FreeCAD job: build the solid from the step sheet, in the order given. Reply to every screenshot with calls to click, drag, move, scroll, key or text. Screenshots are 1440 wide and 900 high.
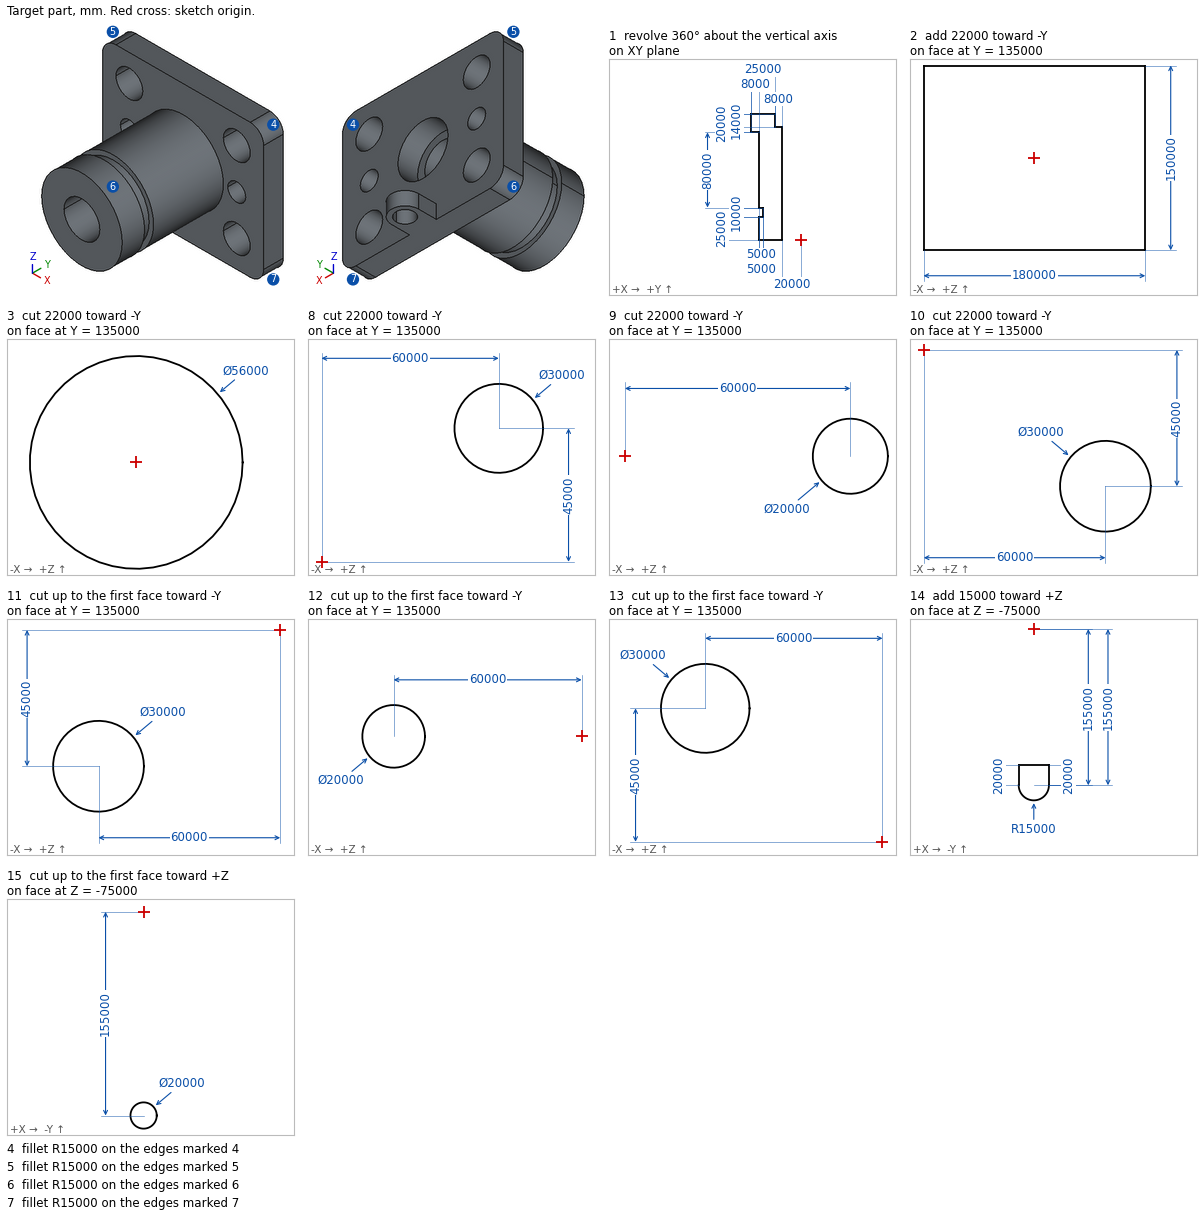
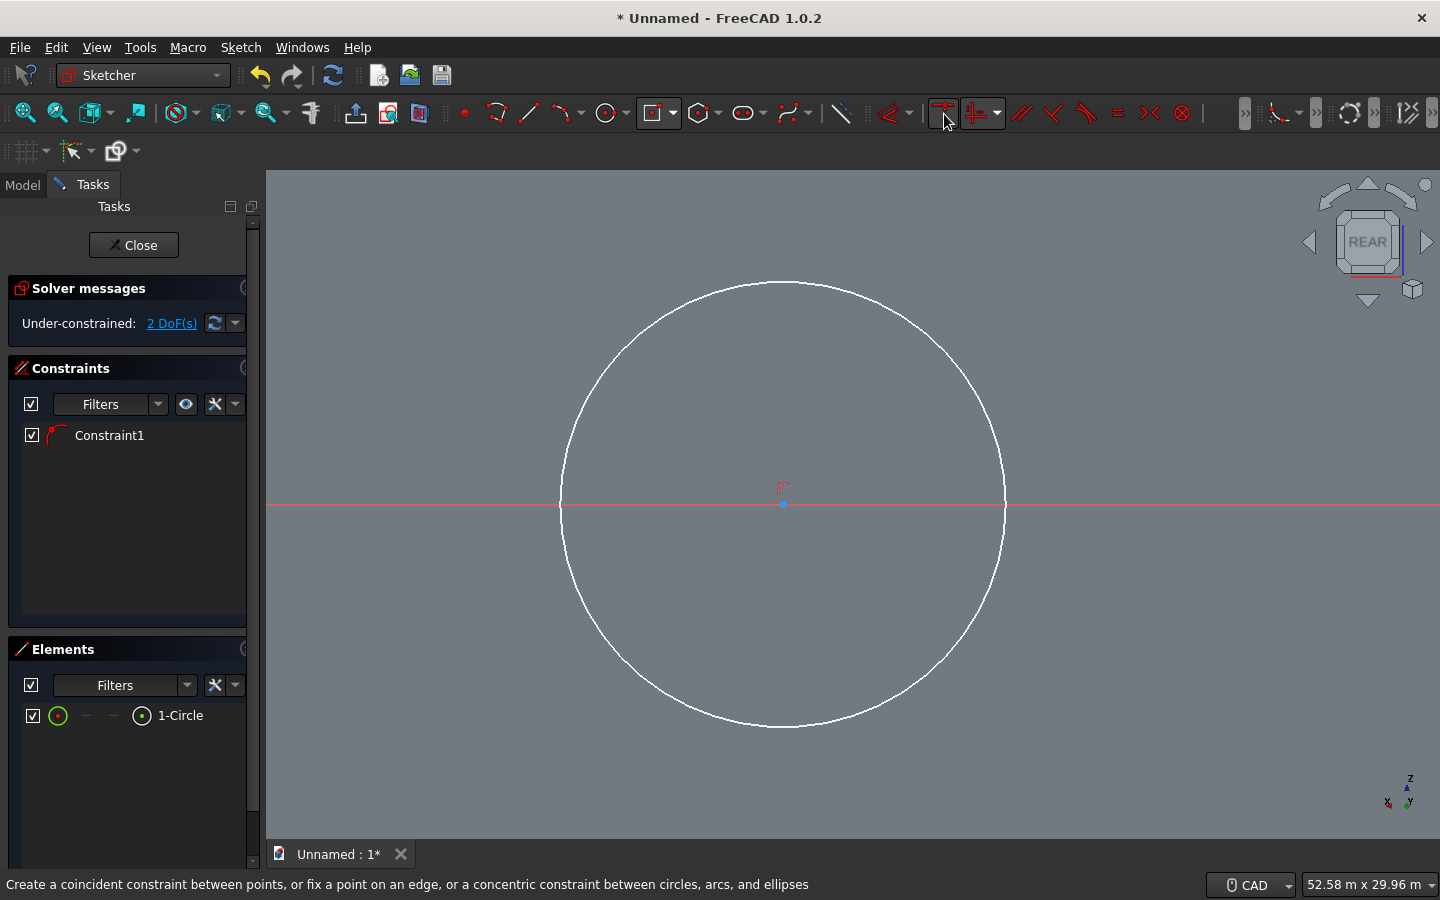
click(940, 347)
click(963, 324)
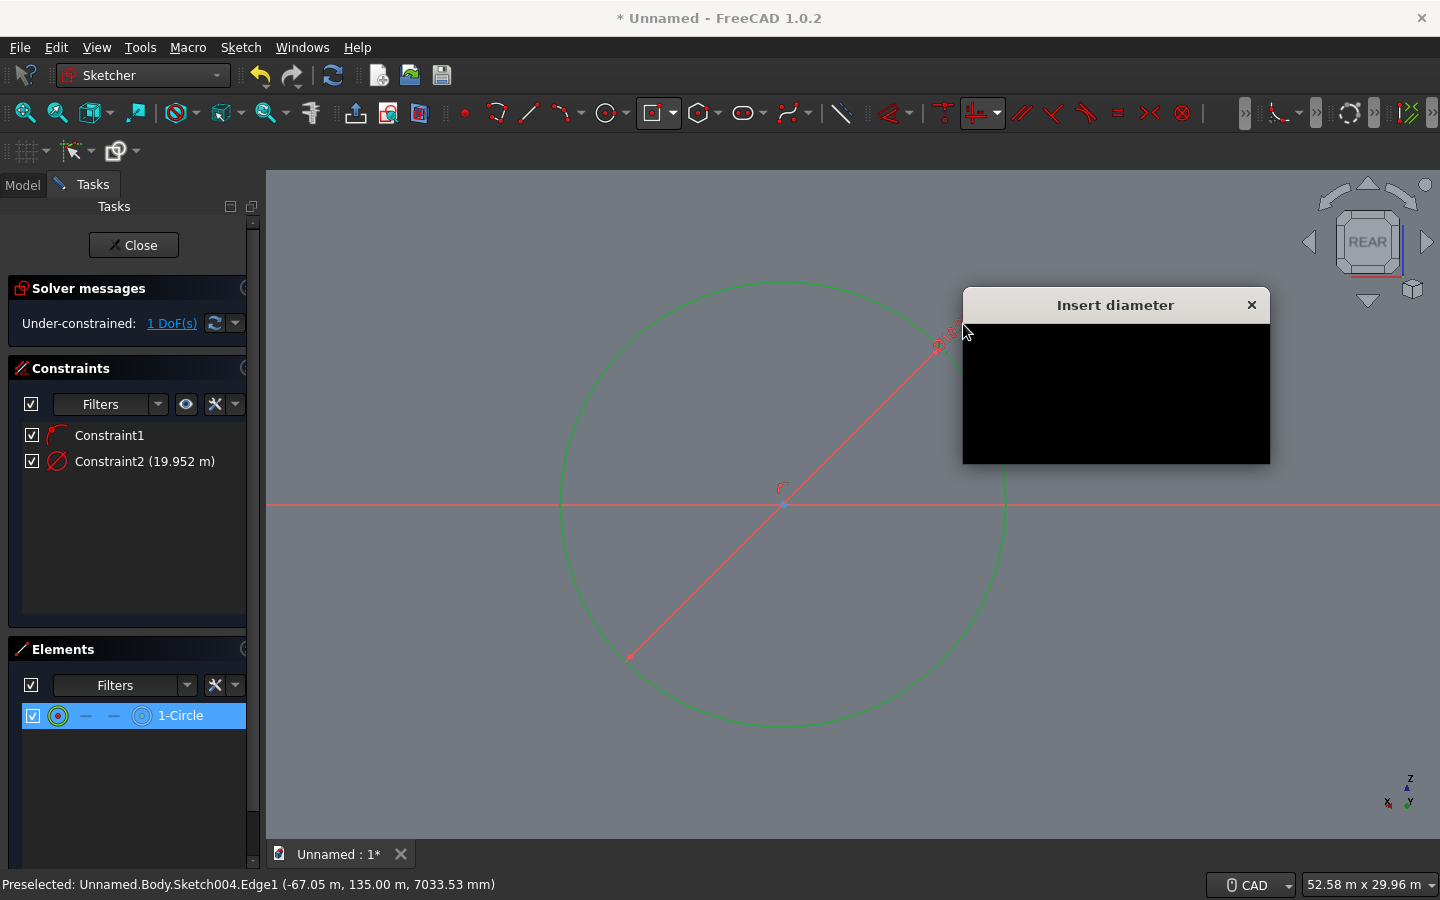
key(ctrl+a)
text(20000 mm)
key(Return)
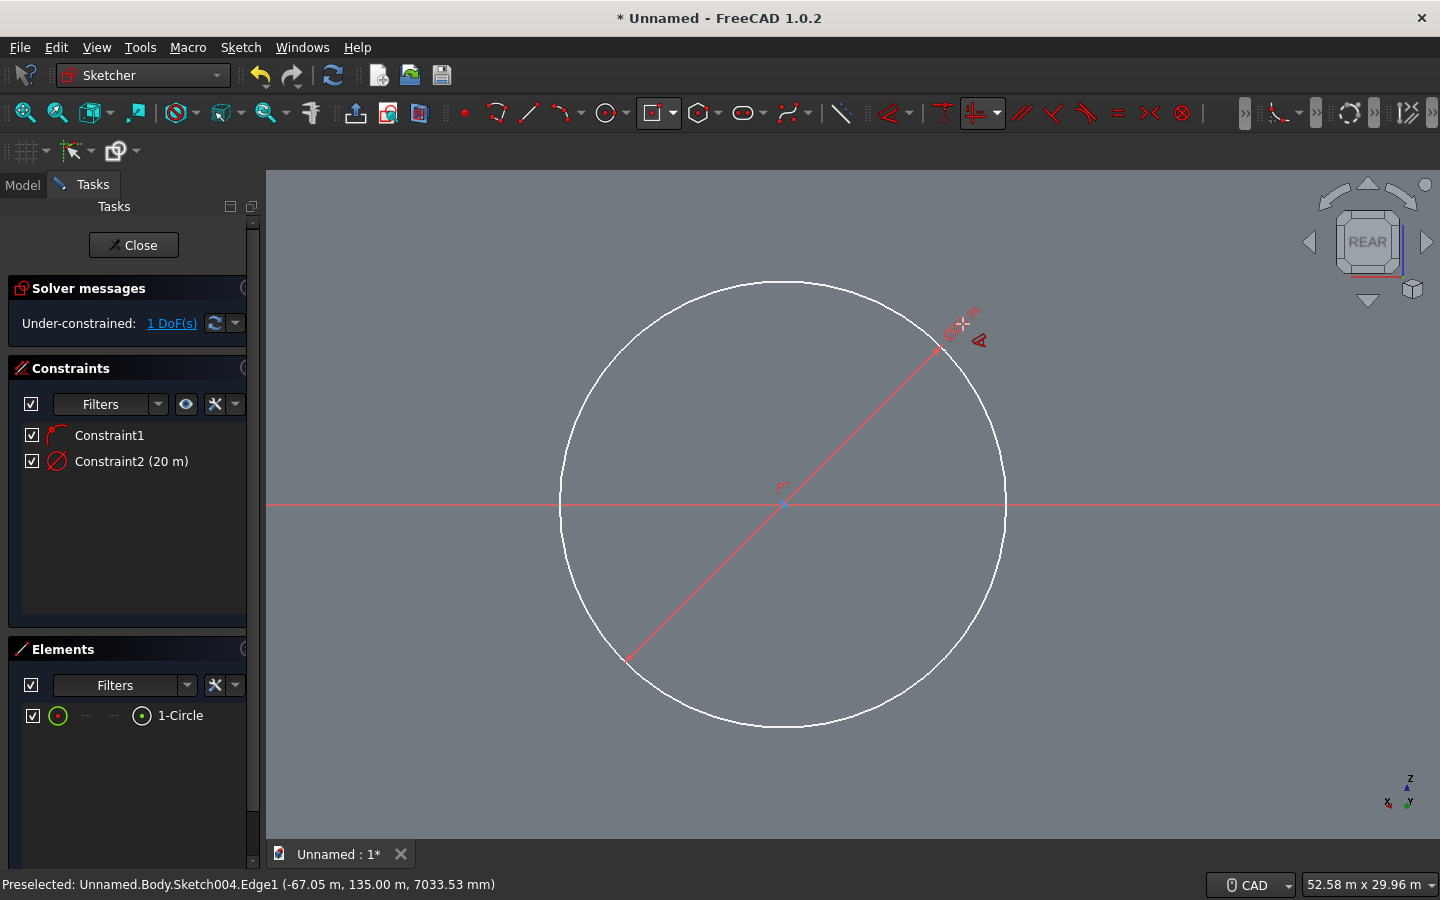
click(783, 504)
click(539, 538)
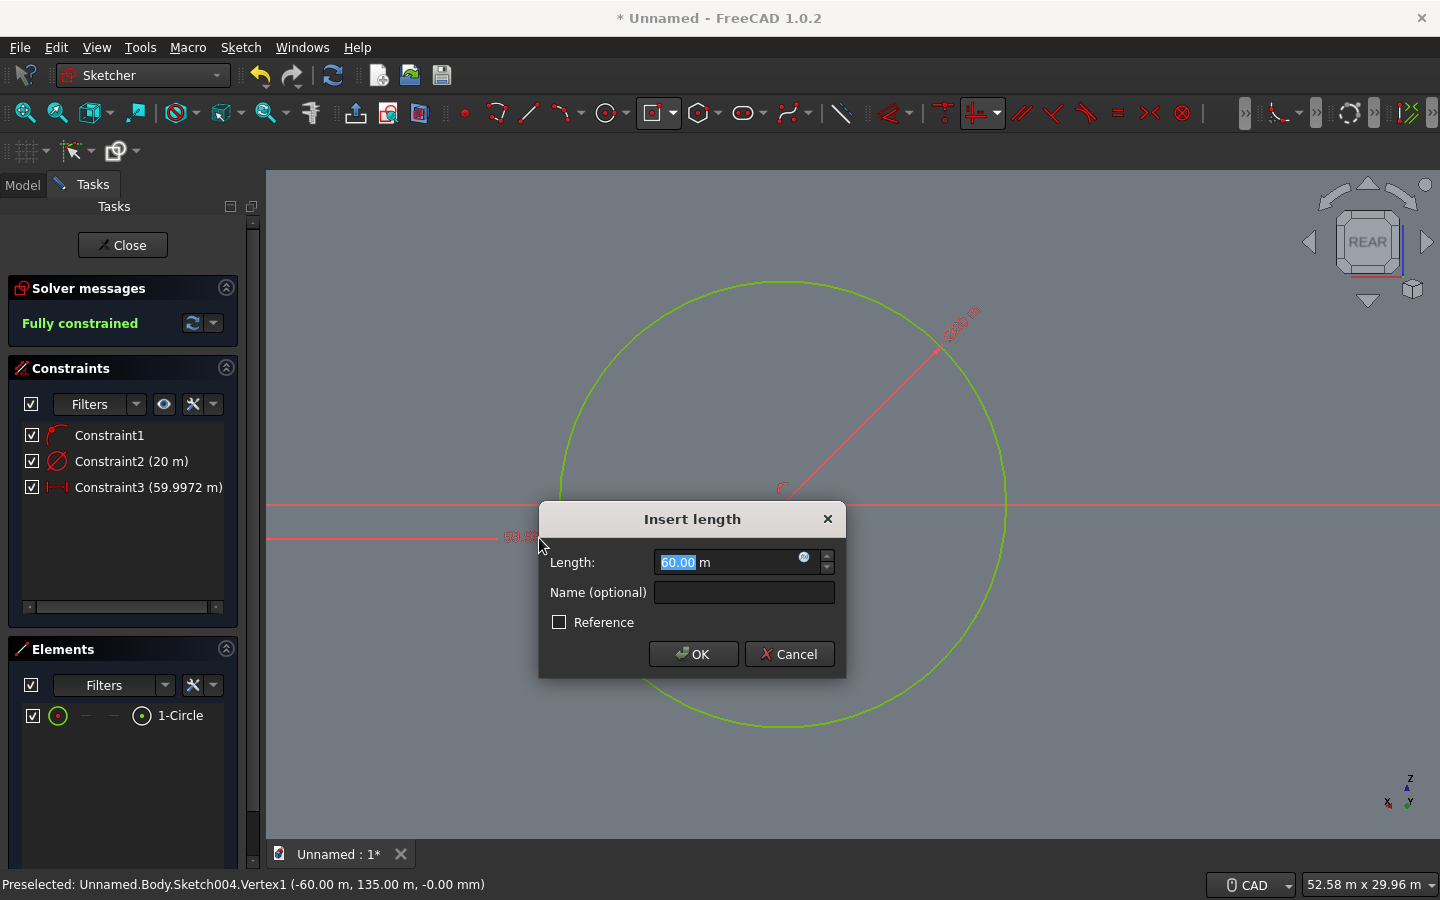
key(ctrl+a)
text(60000 mm)
key(Return)
key(Escape)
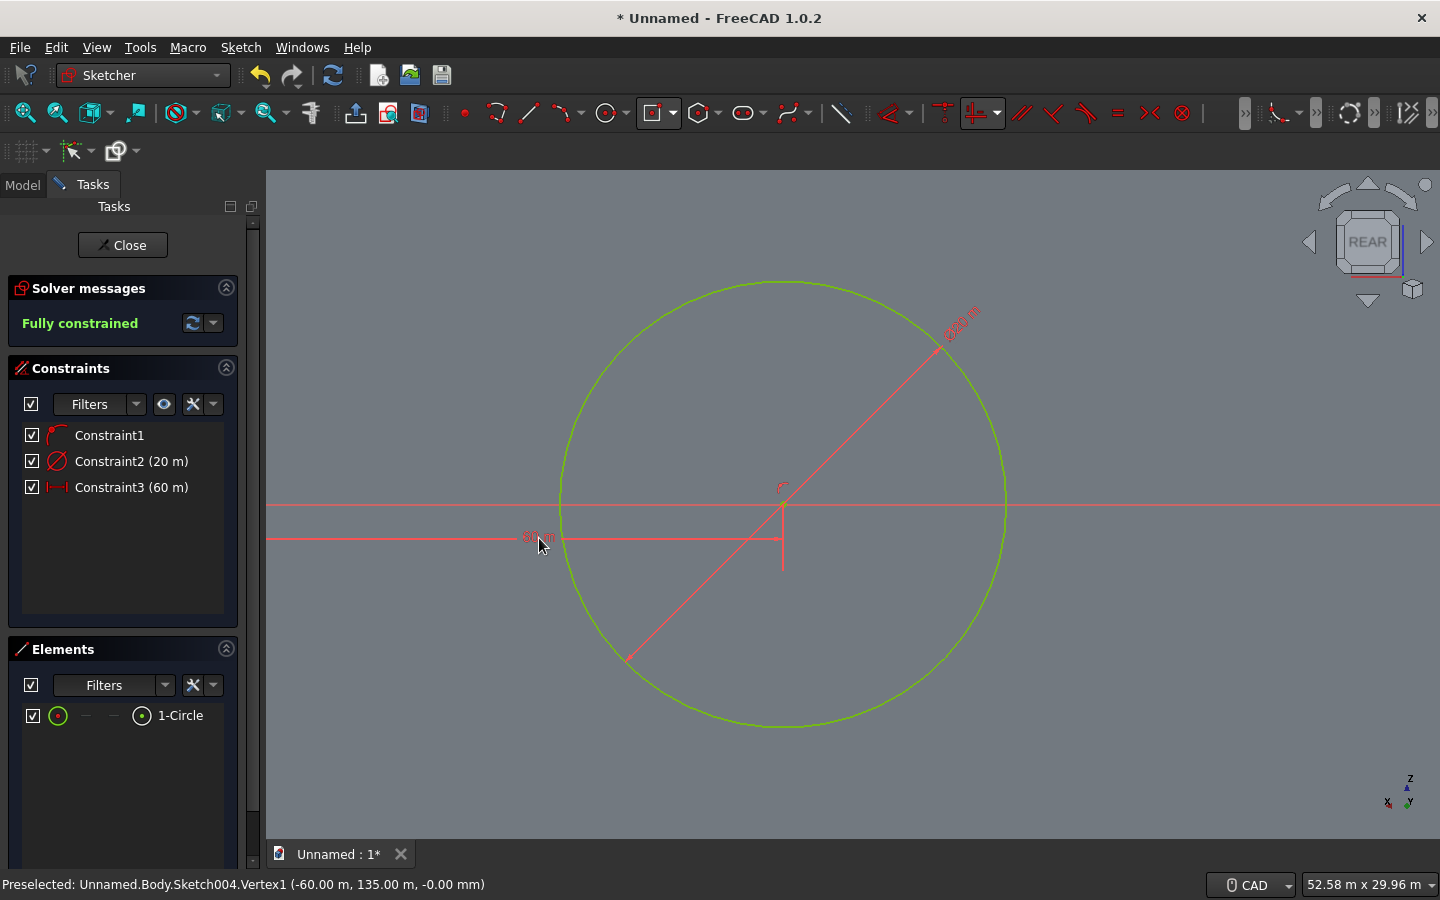
click(123, 245)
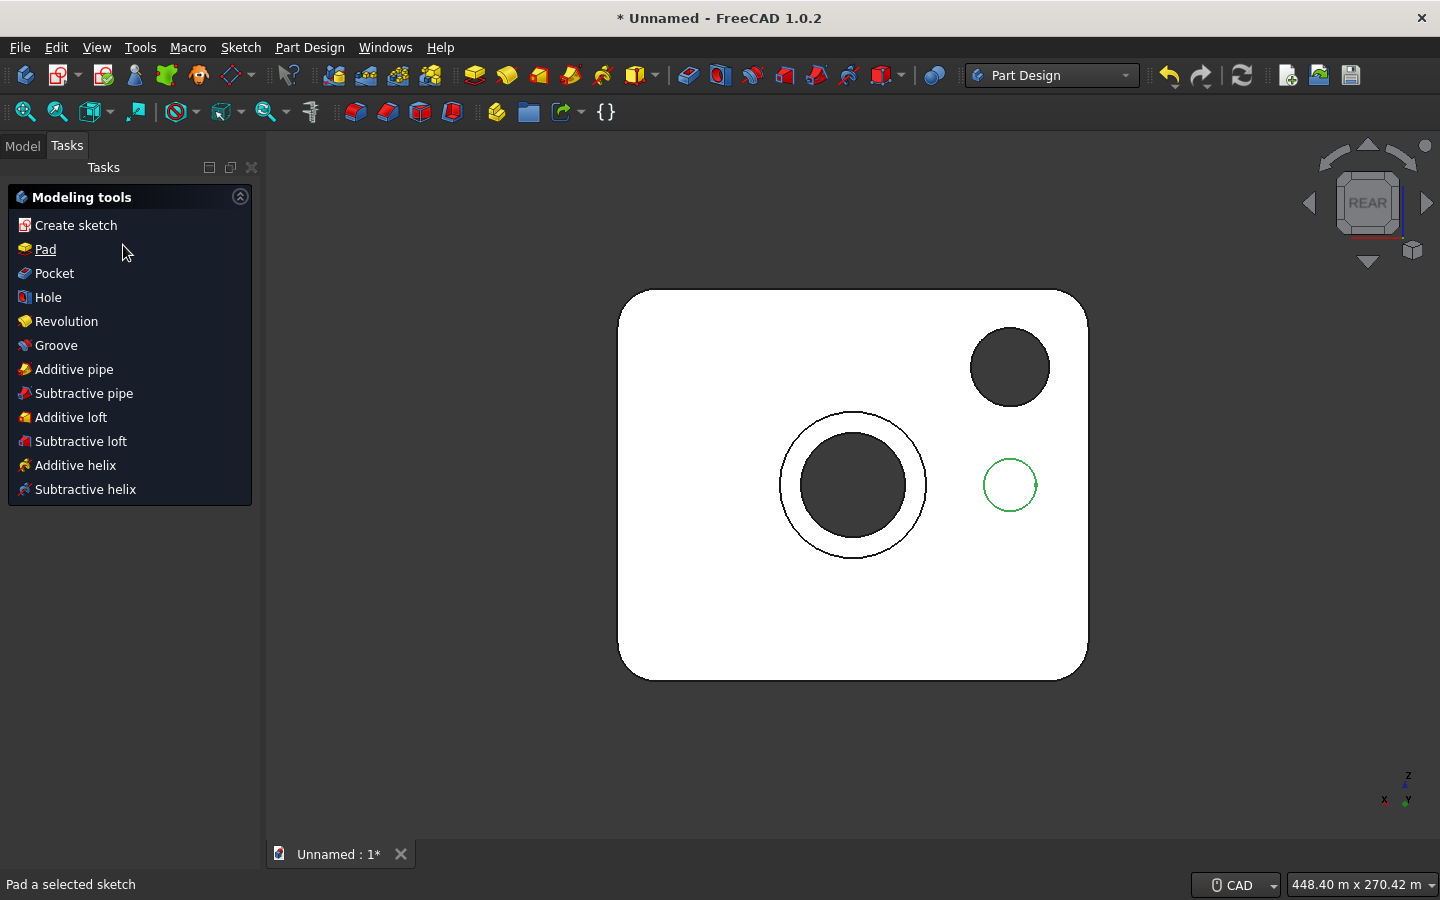
click(690, 76)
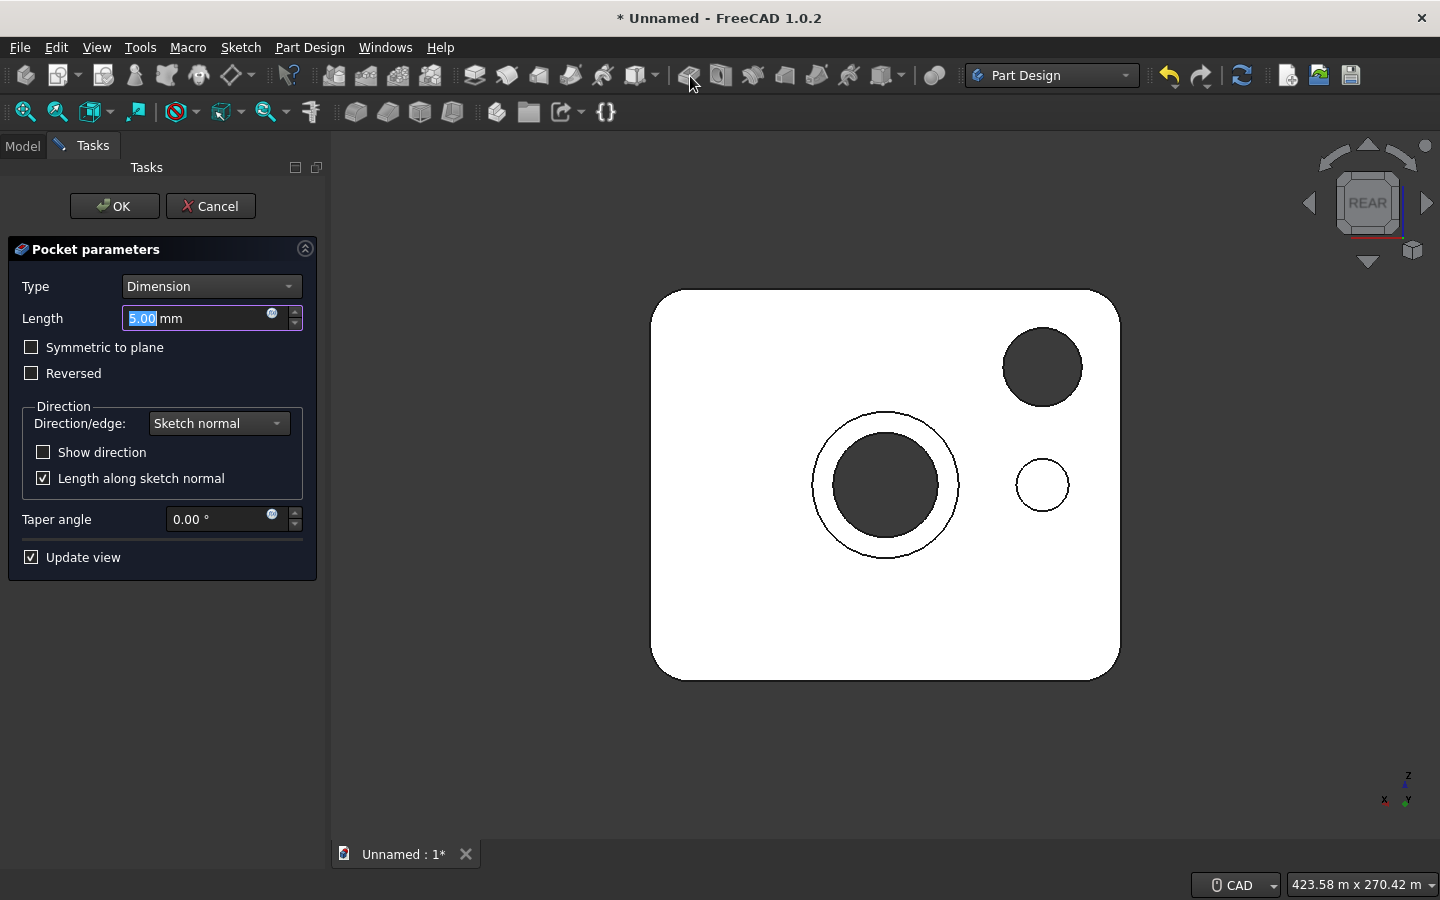
text(22000)
key(Tab)